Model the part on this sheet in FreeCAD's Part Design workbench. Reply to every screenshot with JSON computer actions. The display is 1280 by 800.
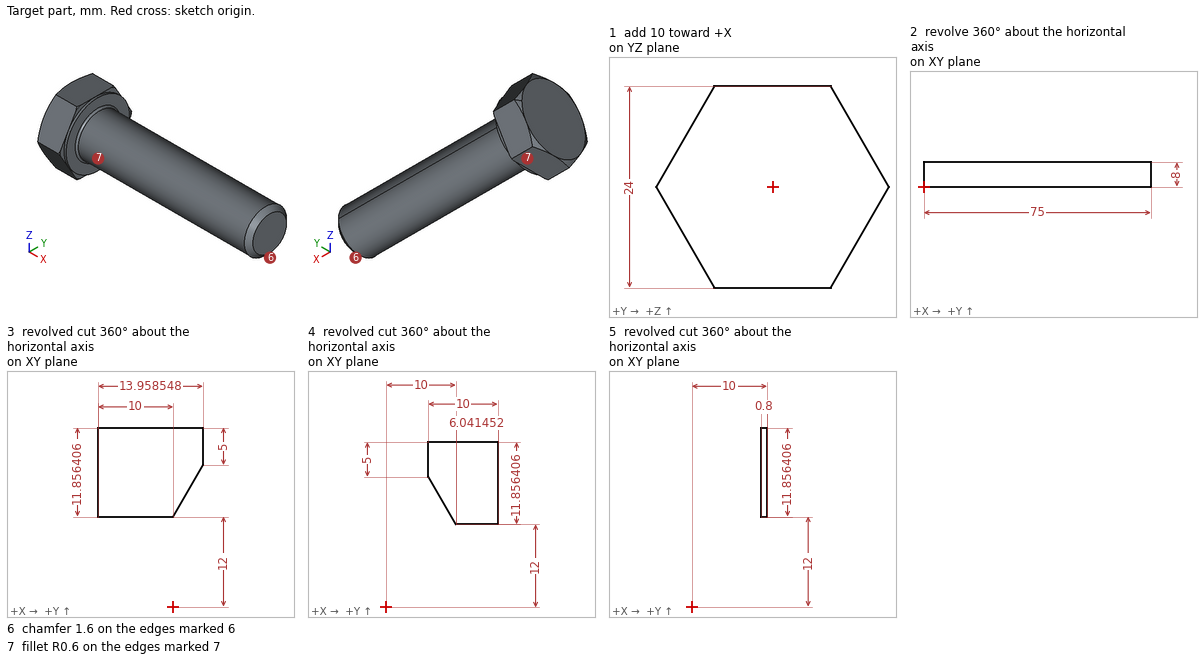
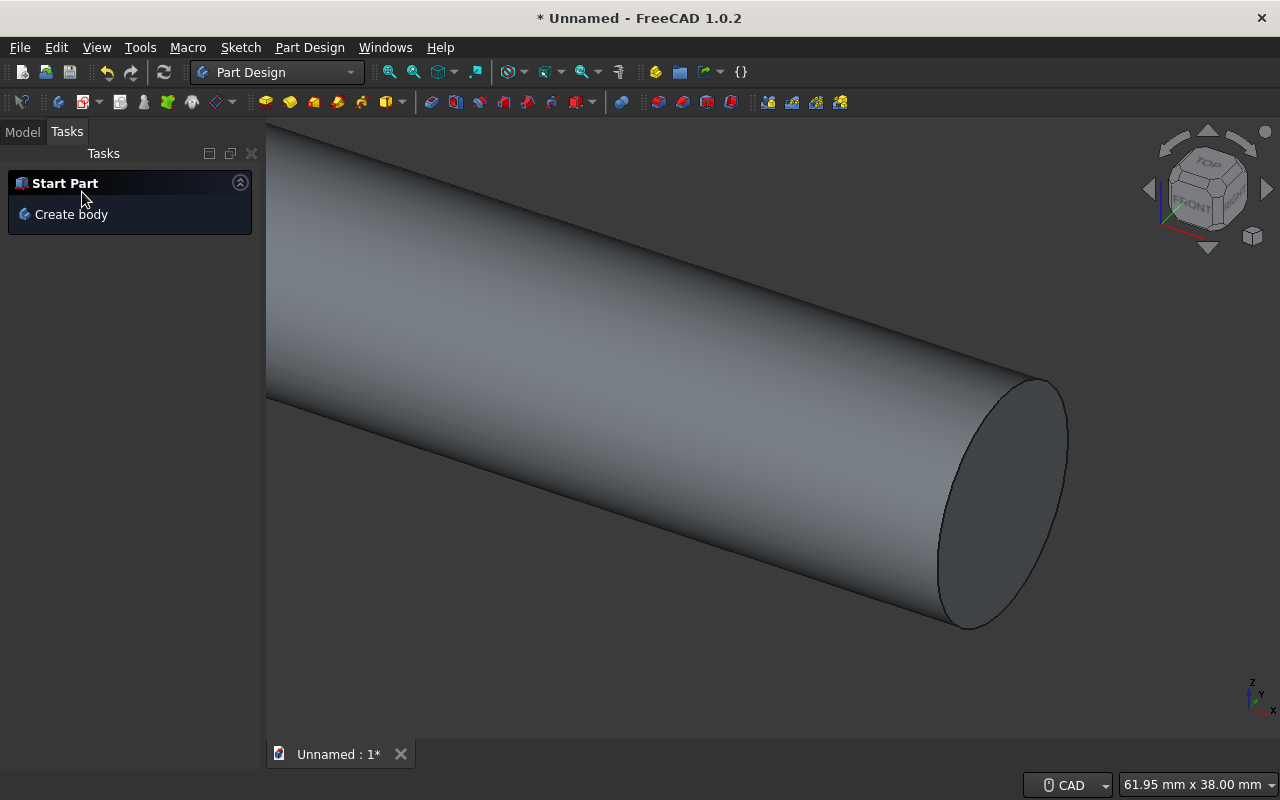
{"action": "left_click", "coordinate": [390, 72]}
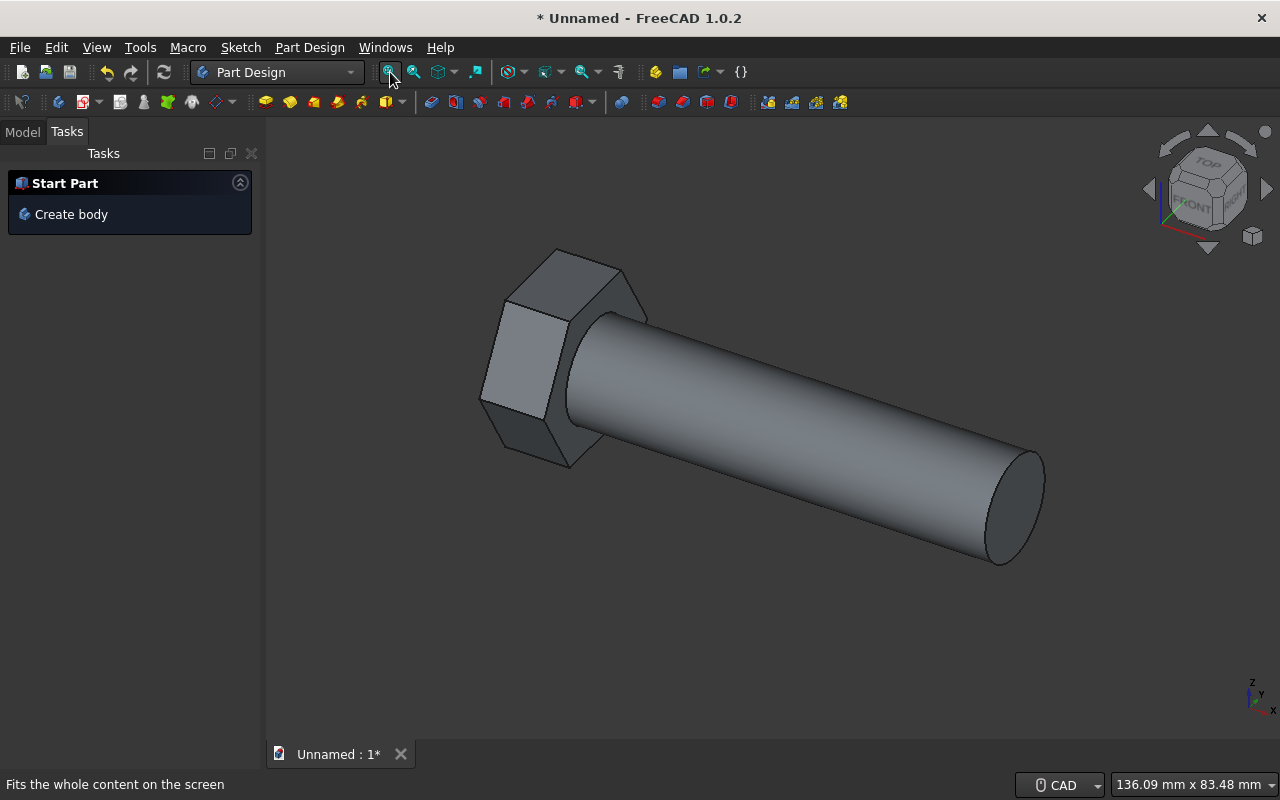
{"action": "left_click", "coordinate": [84, 102]}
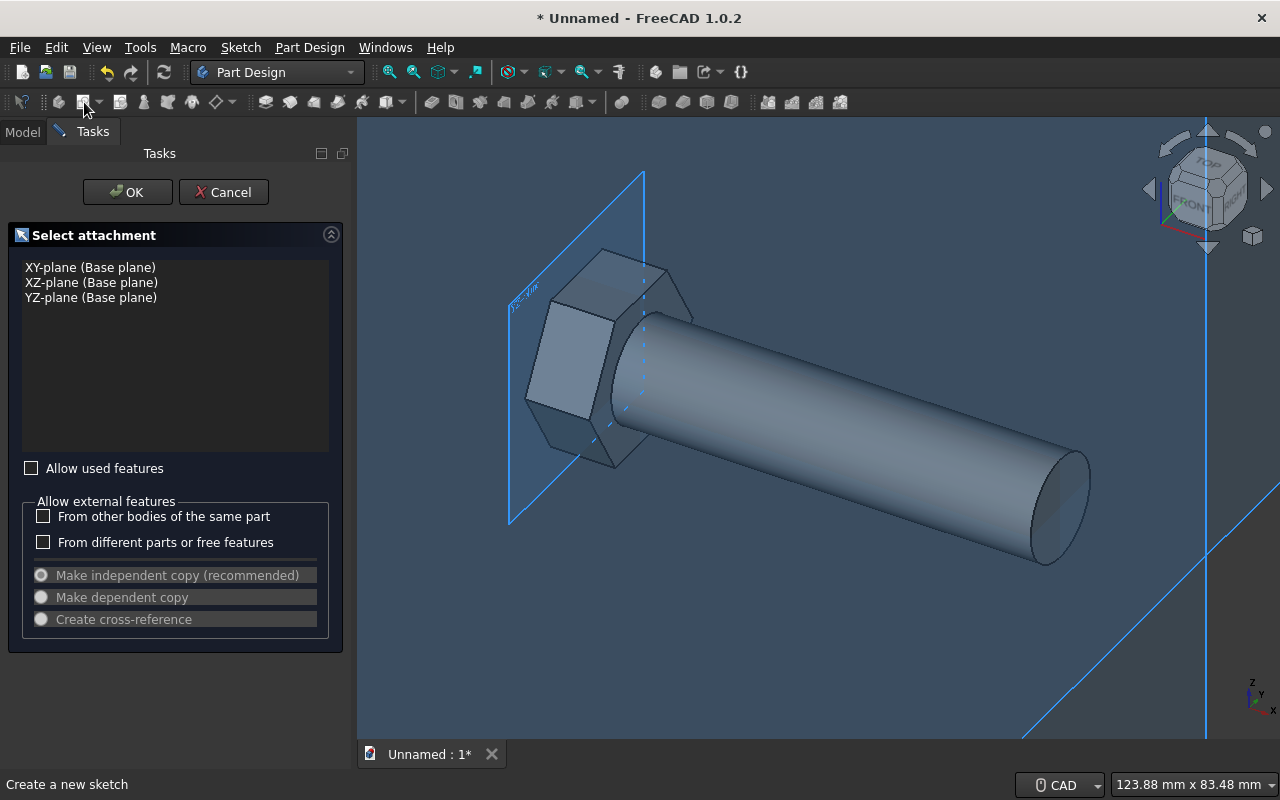
{"action": "left_click", "coordinate": [82, 268]}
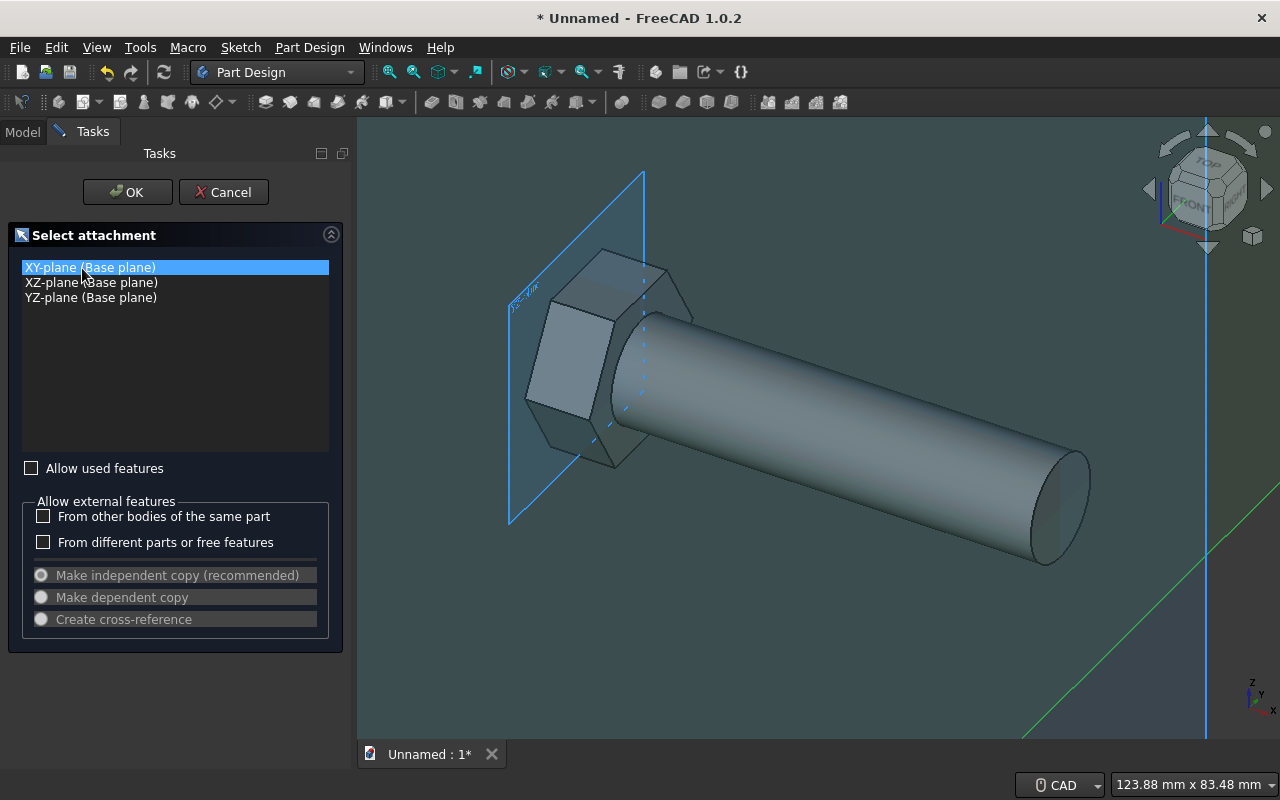
{"action": "left_click", "coordinate": [128, 192]}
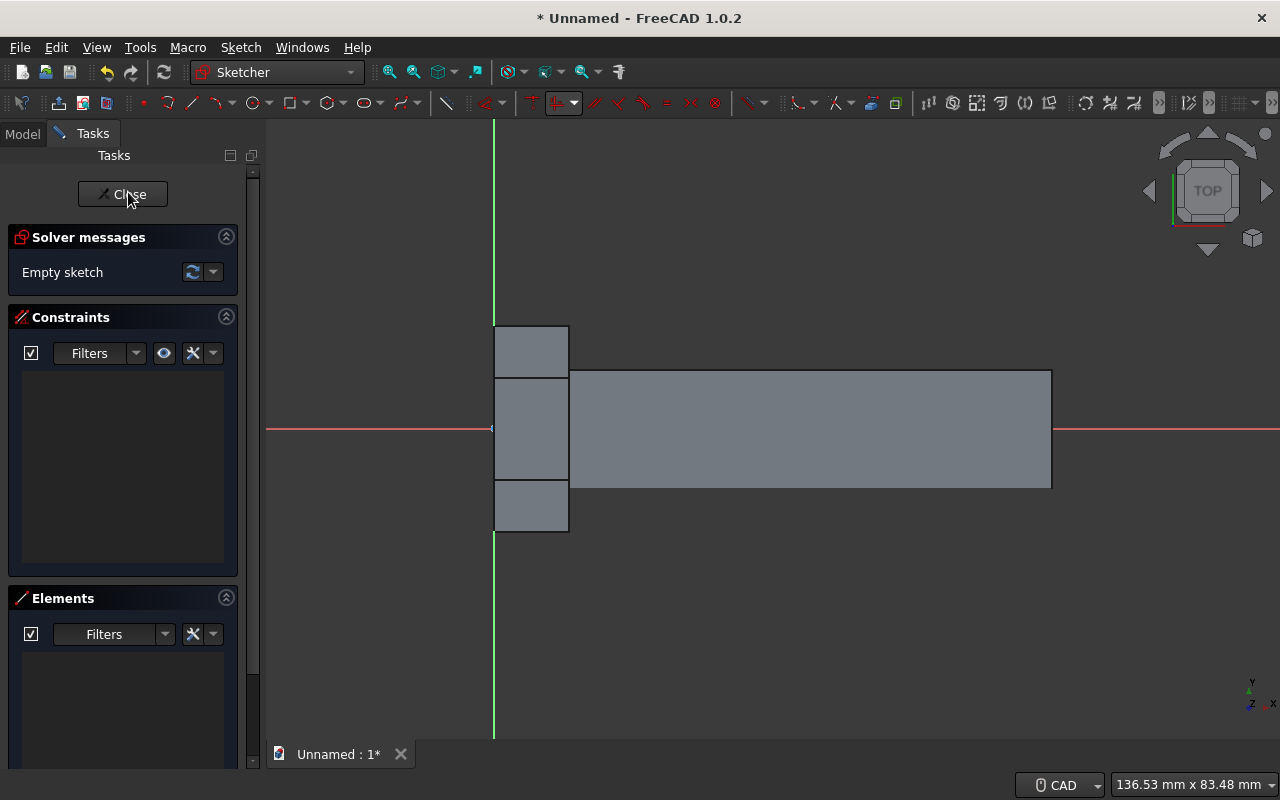
{"action": "left_click", "coordinate": [108, 104]}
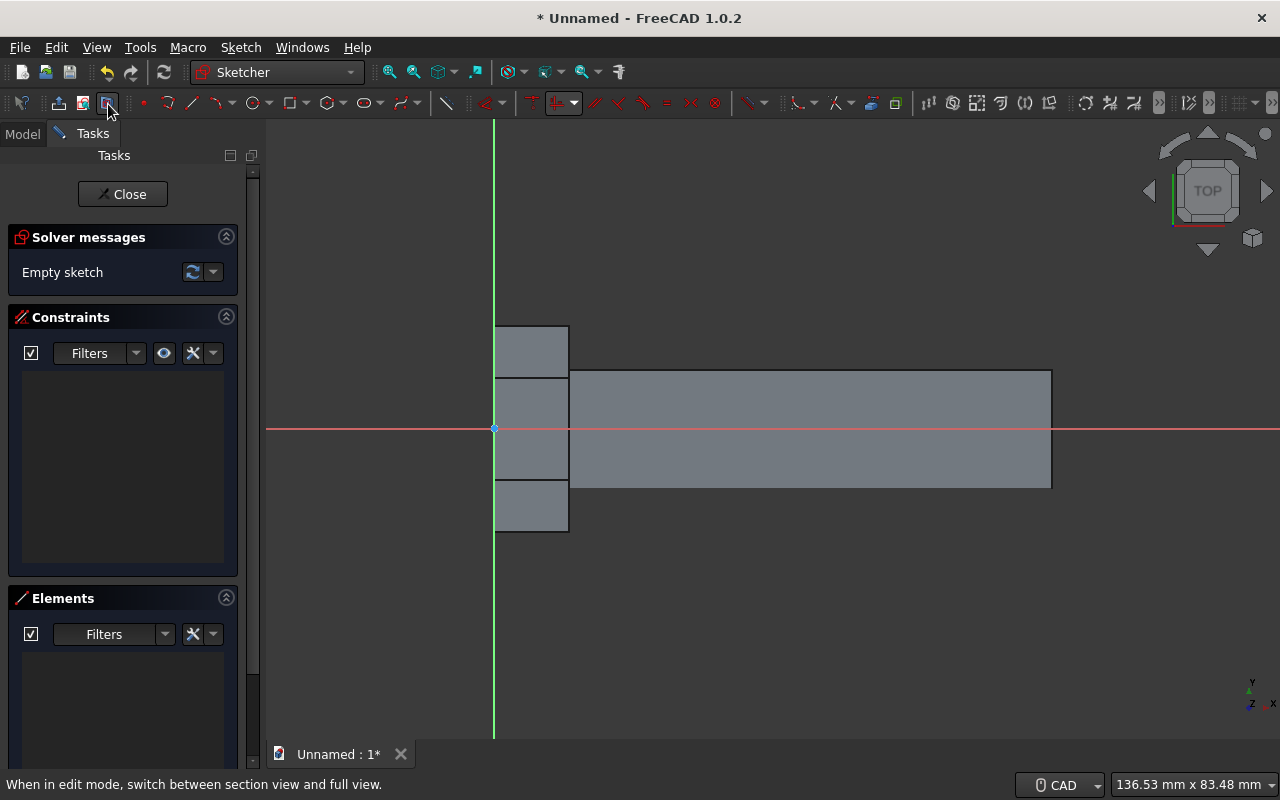
{"action": "scroll", "coordinate": [294, 268], "scroll_direction": "up", "scroll_amount": 4}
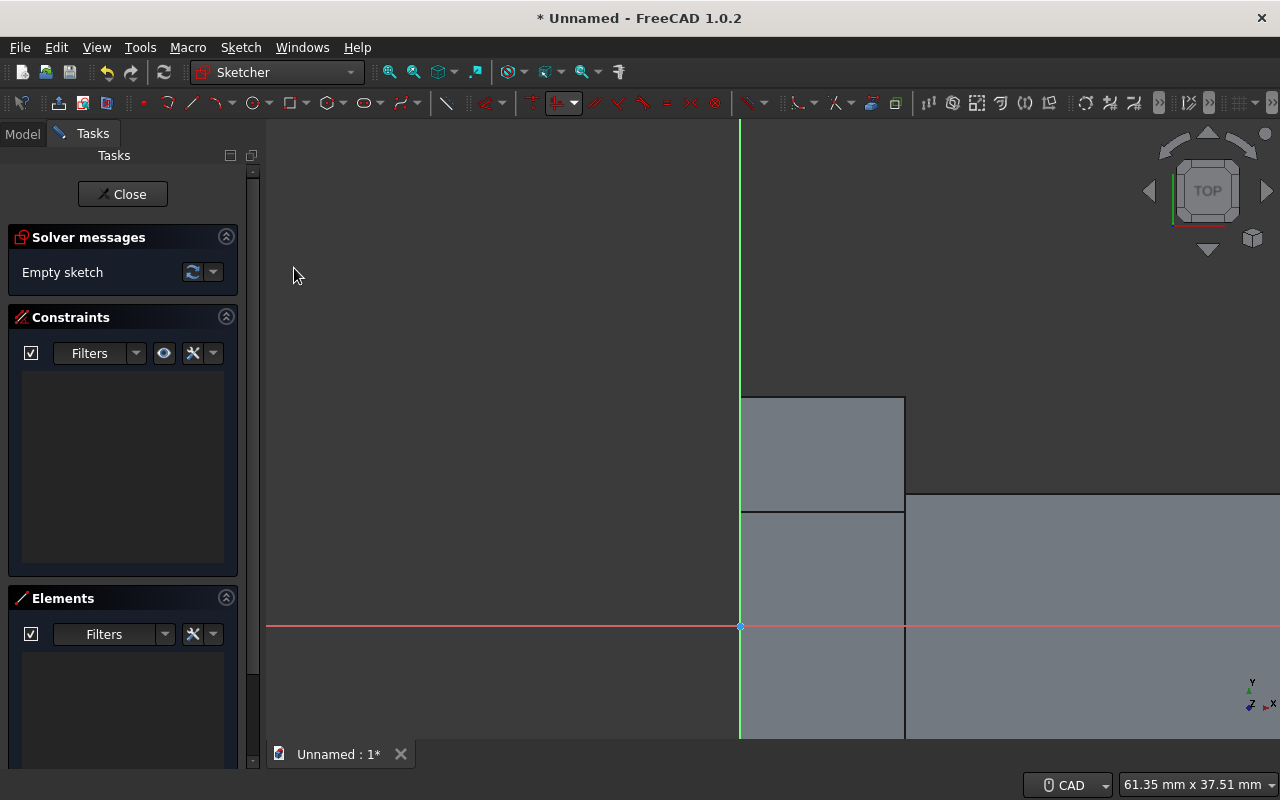
{"action": "left_click", "coordinate": [168, 104]}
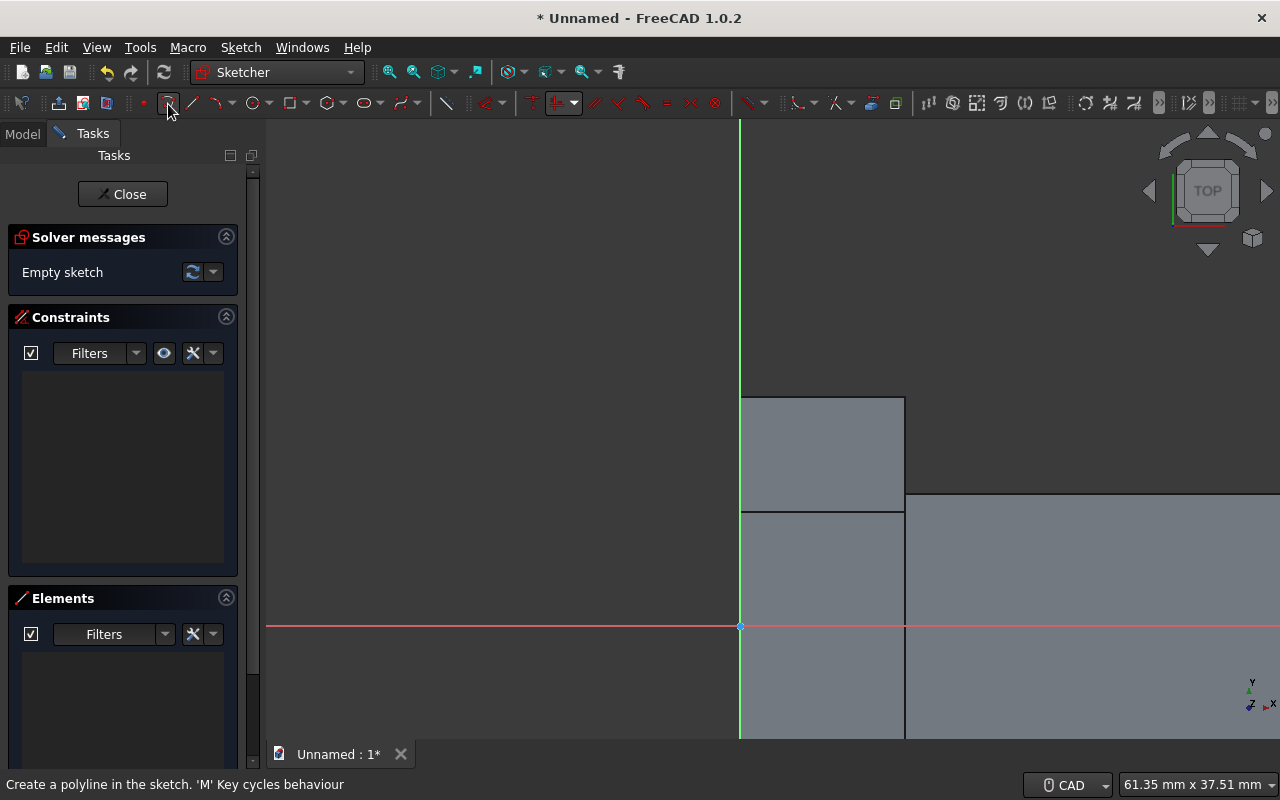
{"action": "left_click", "coordinate": [740, 428]}
{"action": "left_click", "coordinate": [806, 314]}
{"action": "left_click", "coordinate": [806, 232]}
{"action": "left_click", "coordinate": [575, 232]}
{"action": "left_click", "coordinate": [575, 428]}
{"action": "left_click", "coordinate": [740, 429]}
{"action": "key", "text": "Escape"}
{"action": "key", "text": "Escape"}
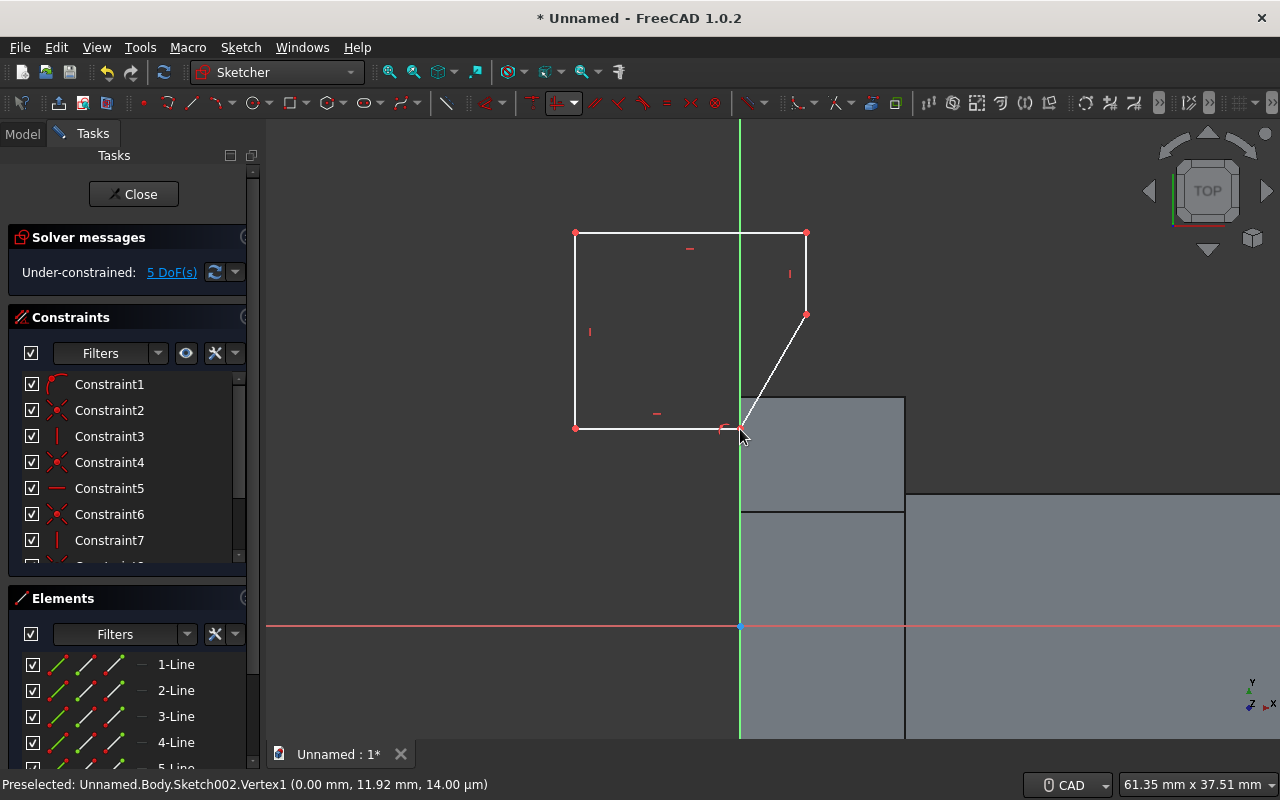
{"action": "left_click", "coordinate": [486, 104]}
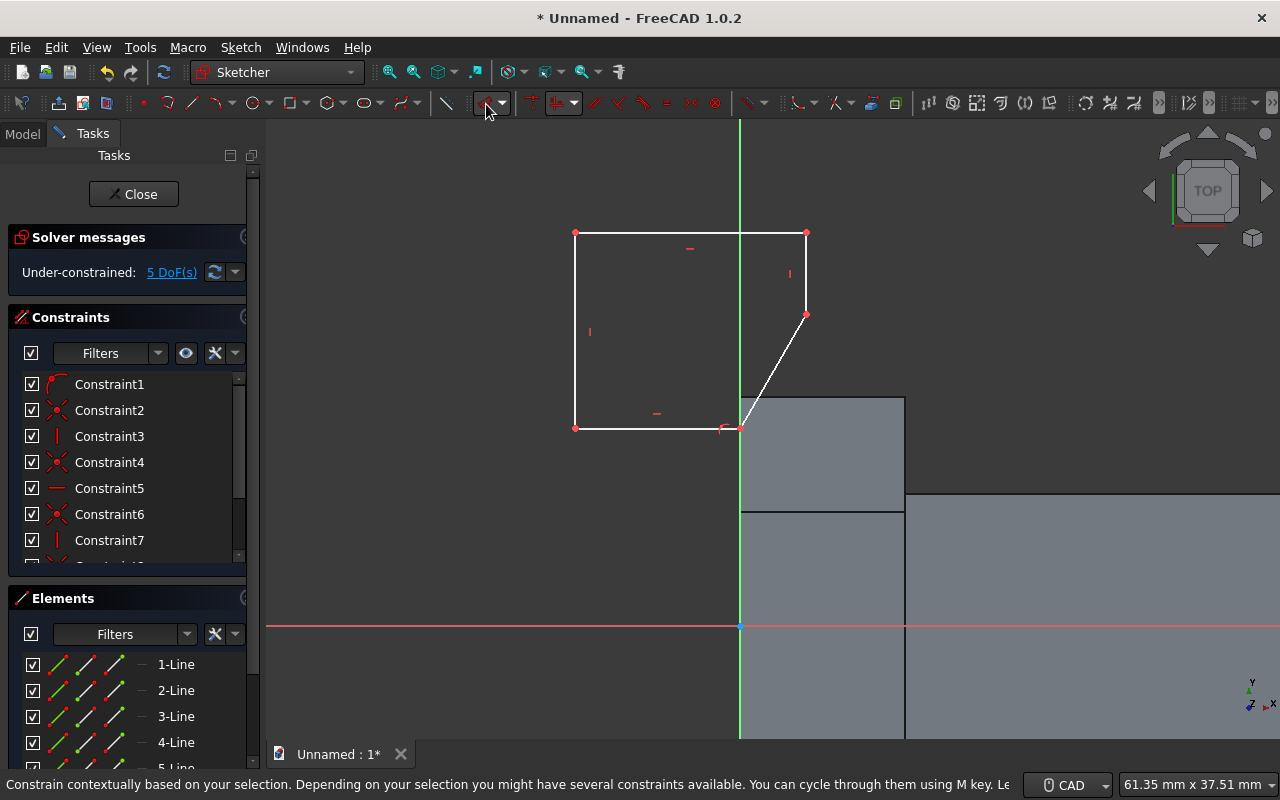
{"action": "left_click", "coordinate": [806, 290]}
{"action": "left_click", "coordinate": [840, 274]}